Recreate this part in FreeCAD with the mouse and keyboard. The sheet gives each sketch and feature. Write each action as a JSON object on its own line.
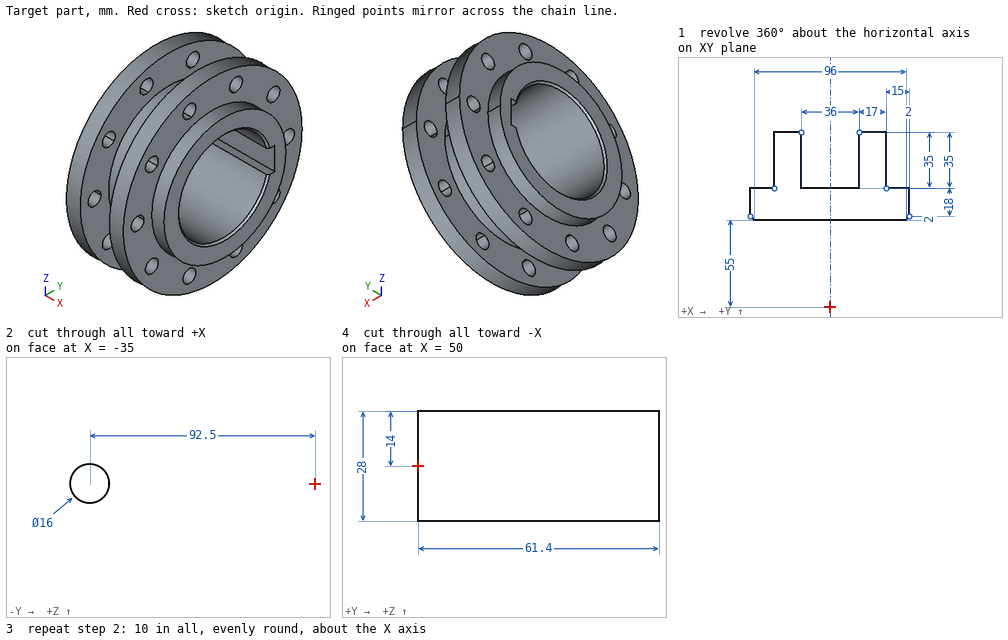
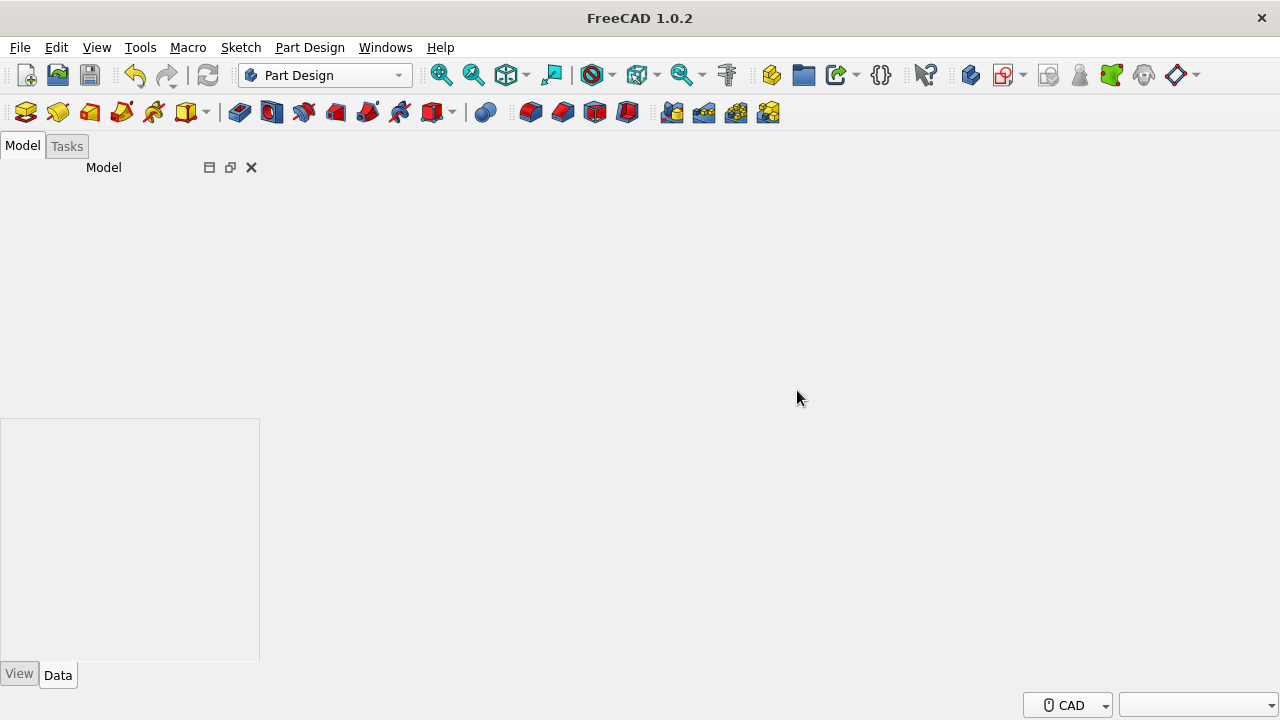
{"action": "left_click", "coordinate": [26, 76]}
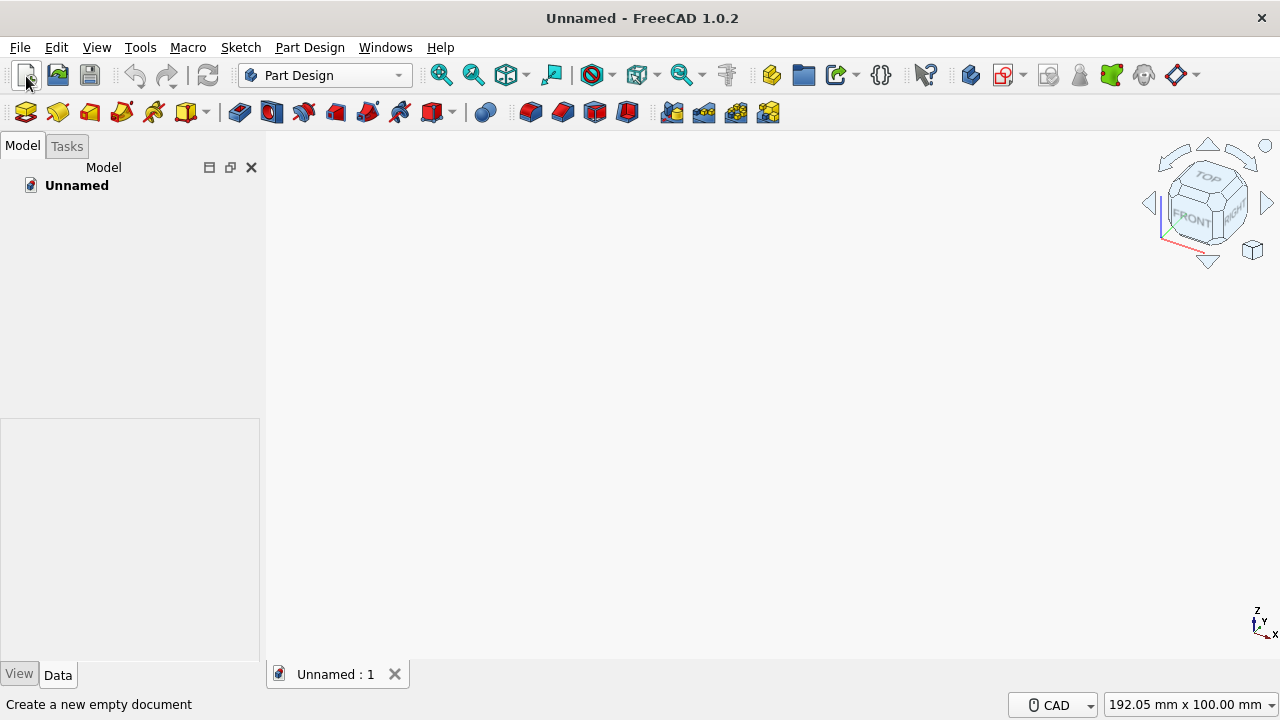
{"action": "left_click", "coordinate": [1004, 76]}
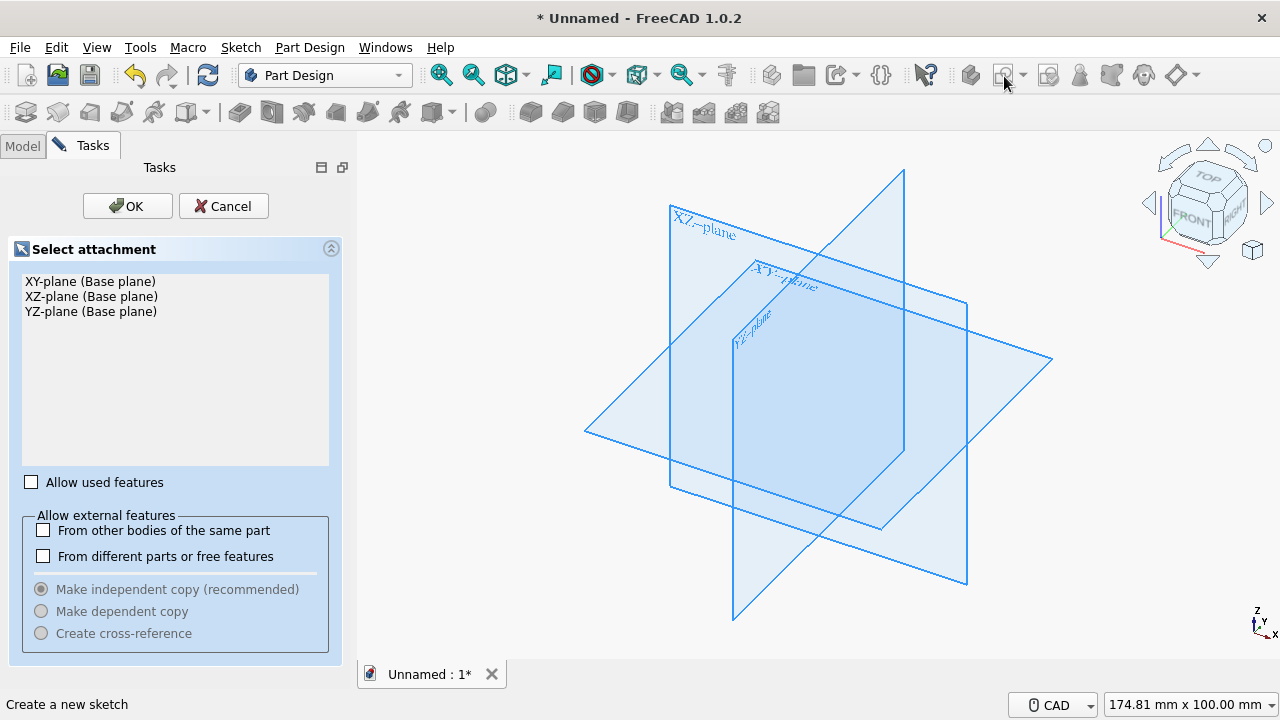
{"action": "left_click", "coordinate": [82, 282]}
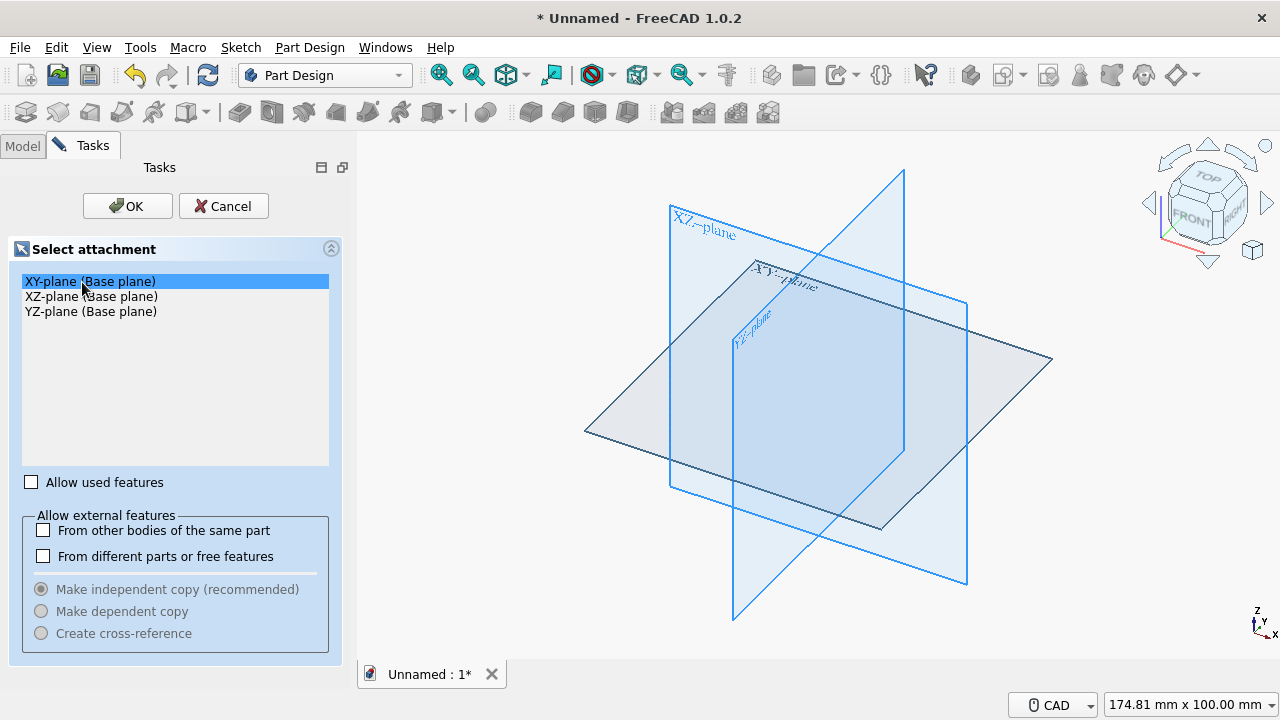
{"action": "left_click", "coordinate": [128, 206]}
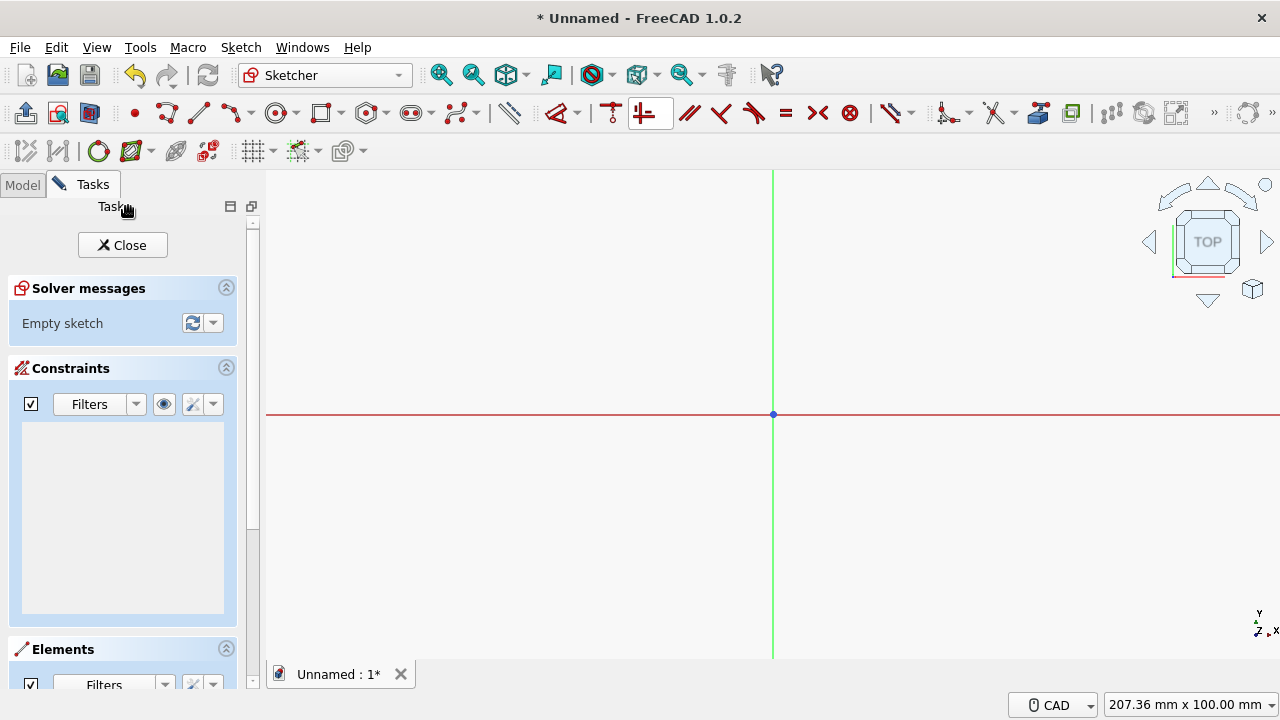
{"action": "scroll", "coordinate": [649, 631], "scroll_direction": "down", "scroll_amount": 4}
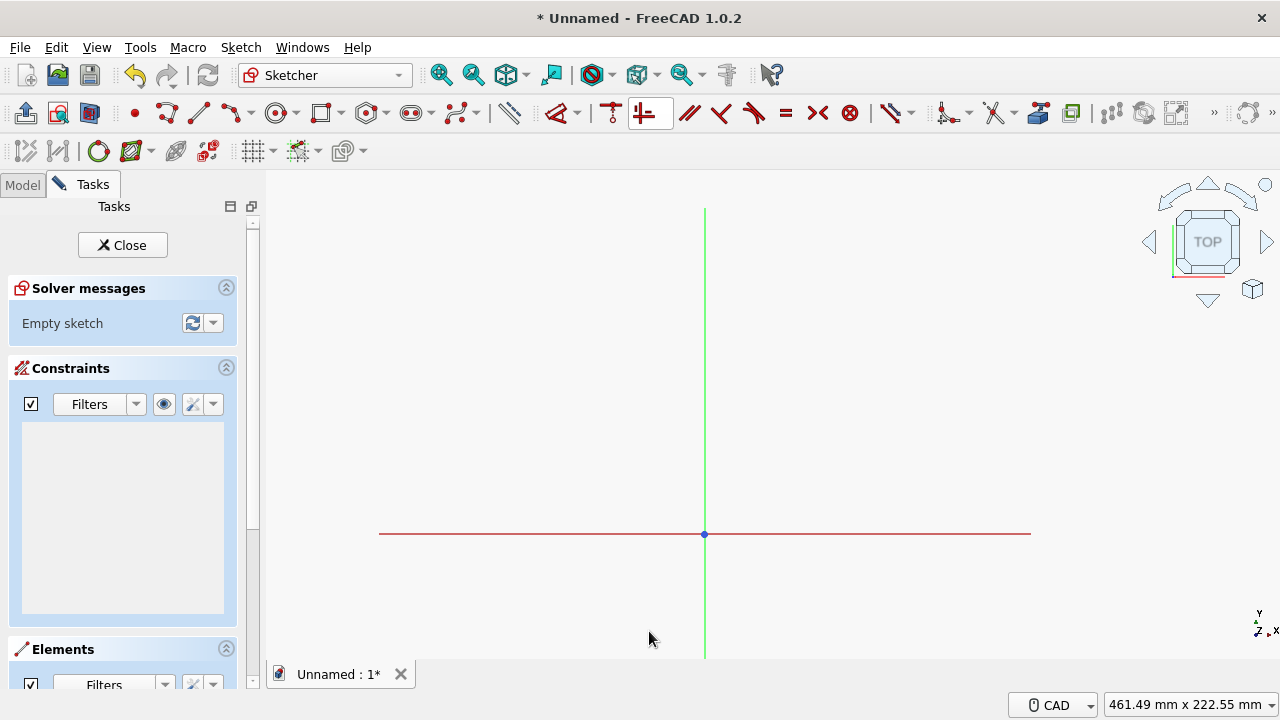
{"action": "left_click", "coordinate": [168, 114]}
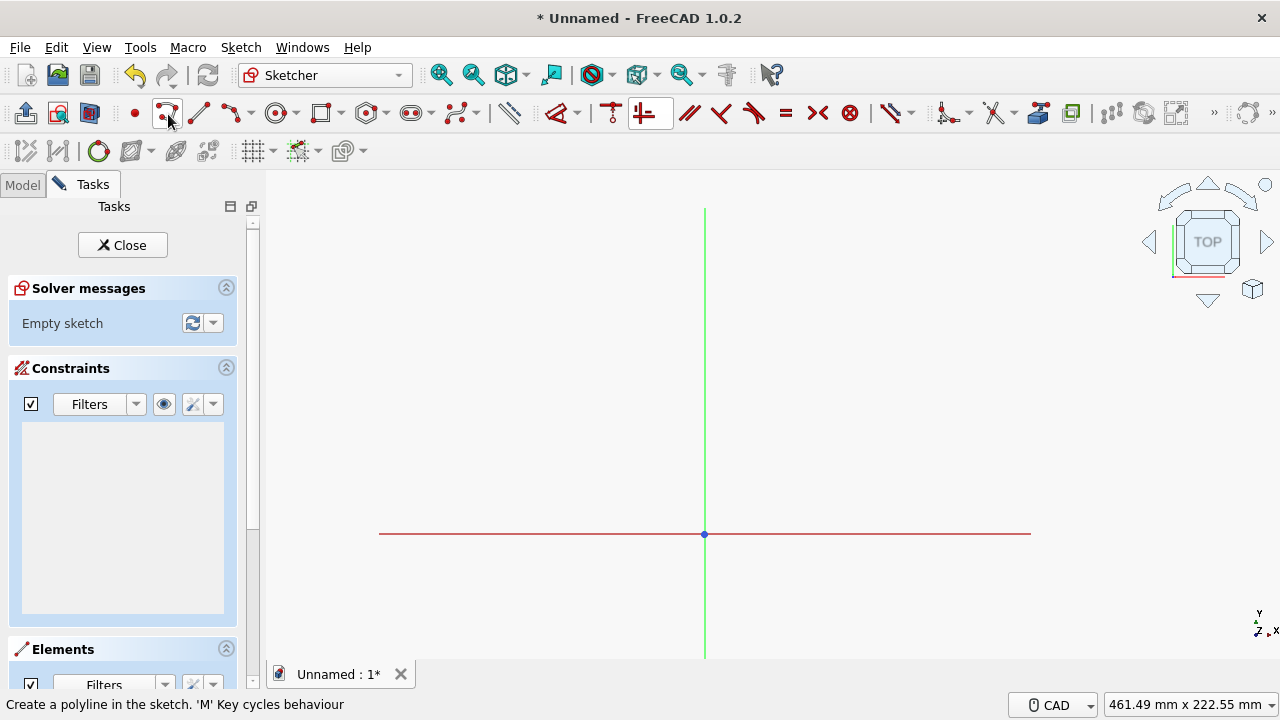
{"action": "left_click", "coordinate": [599, 413]}
{"action": "left_click", "coordinate": [810, 413]}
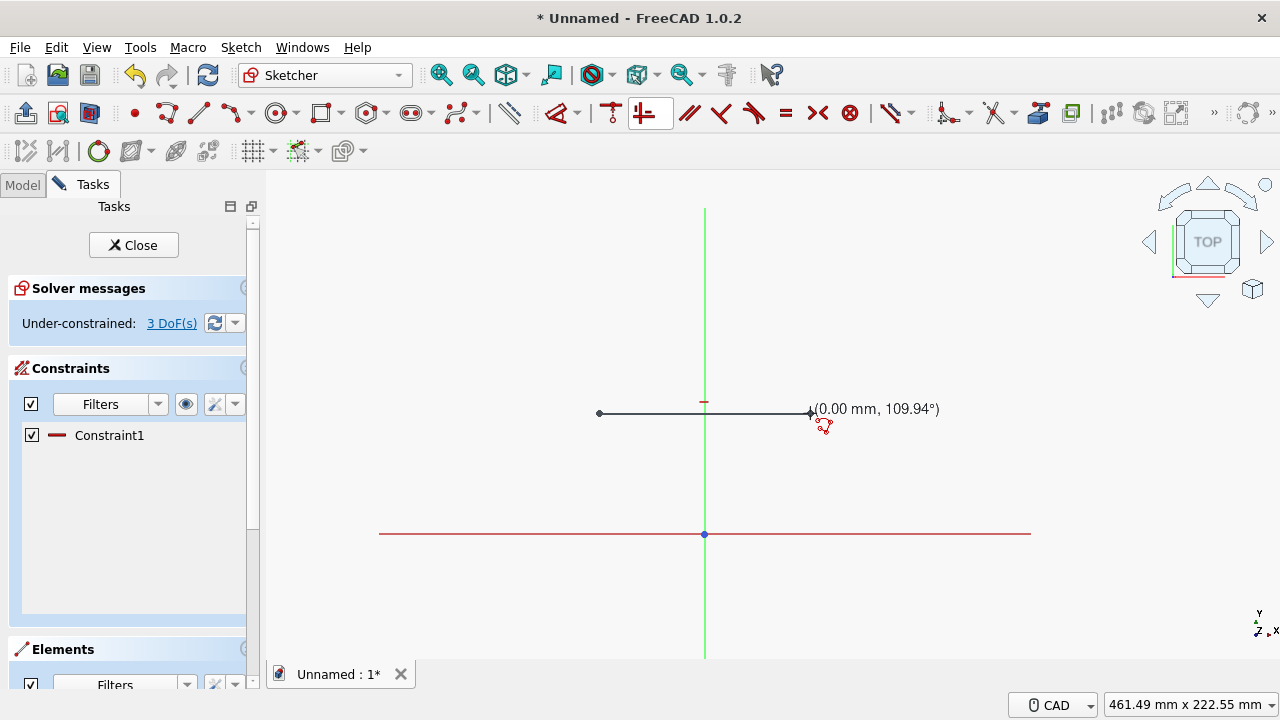
{"action": "scroll", "coordinate": [815, 409], "scroll_direction": "up", "scroll_amount": 5}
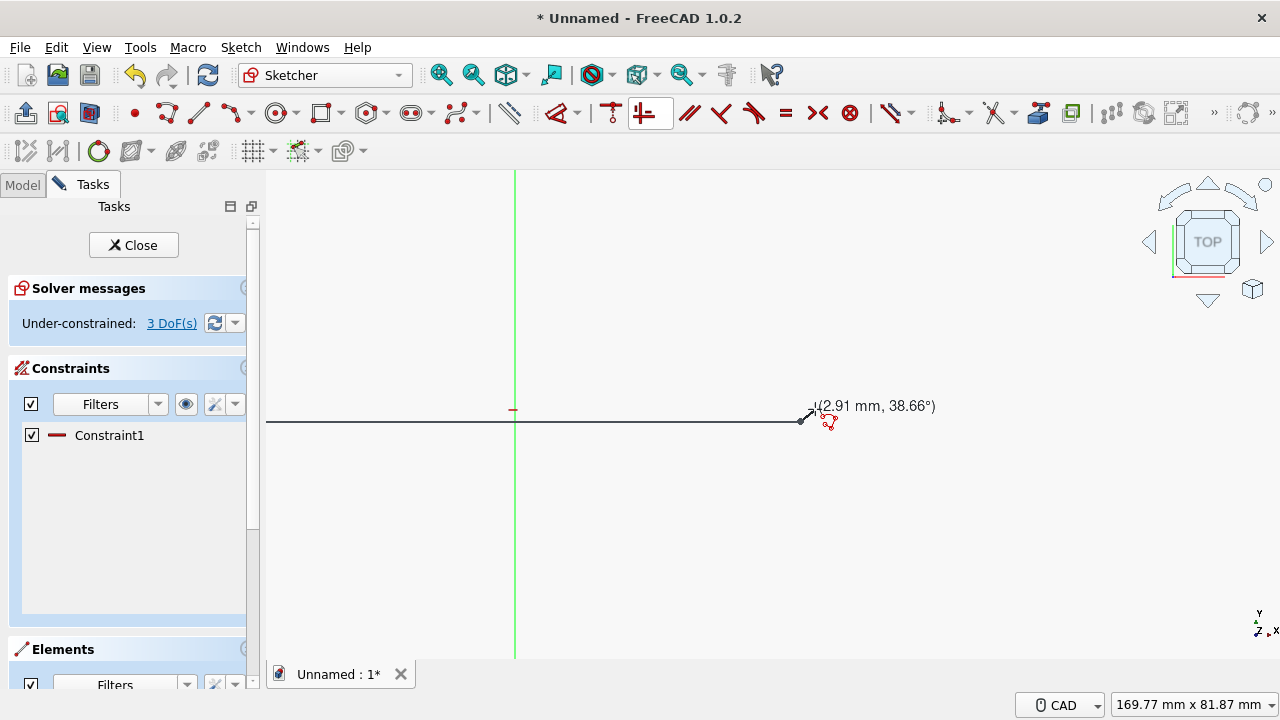
{"action": "left_click", "coordinate": [813, 408]}
{"action": "left_click", "coordinate": [813, 301]}
{"action": "left_click", "coordinate": [724, 301]}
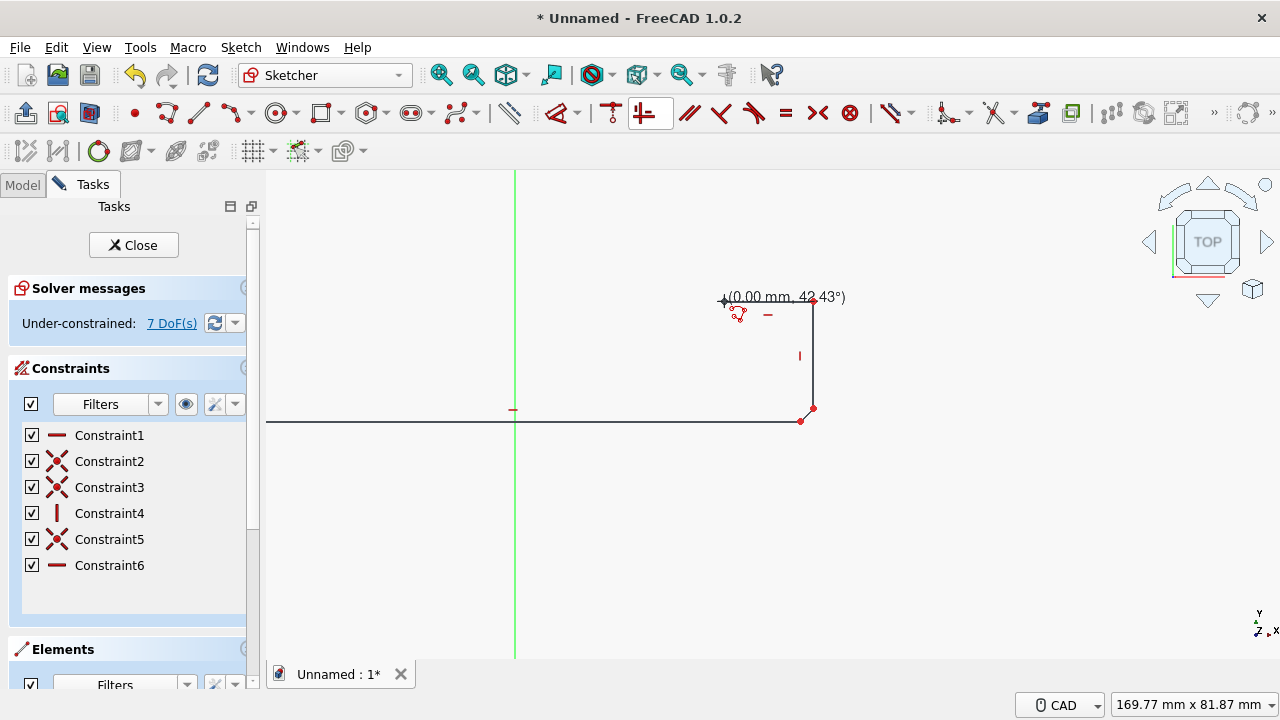
{"action": "scroll", "coordinate": [859, 410], "scroll_direction": "down", "scroll_amount": 4}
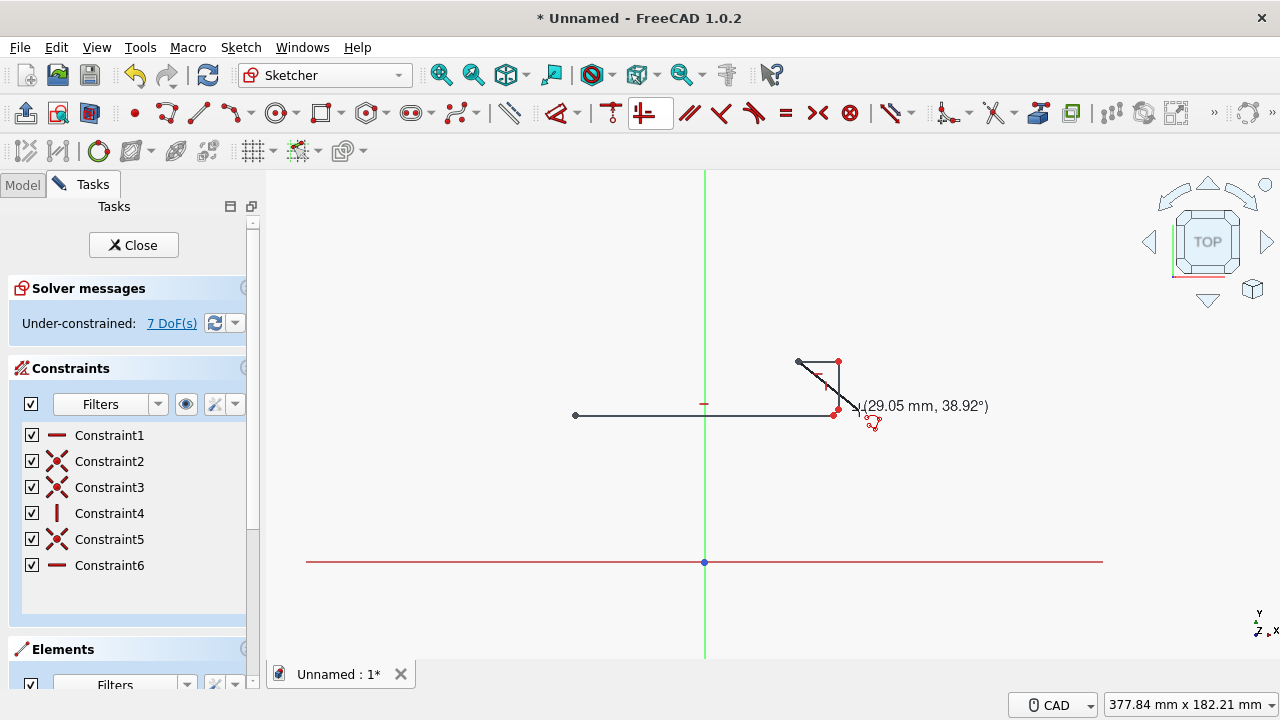
{"action": "left_click", "coordinate": [799, 267]}
{"action": "left_click", "coordinate": [753, 267]}
{"action": "left_click", "coordinate": [753, 361]}
{"action": "left_click", "coordinate": [656, 361]}
{"action": "left_click", "coordinate": [656, 267]}
{"action": "left_click", "coordinate": [611, 267]}
{"action": "left_click", "coordinate": [611, 361]}
{"action": "left_click", "coordinate": [571, 361]}